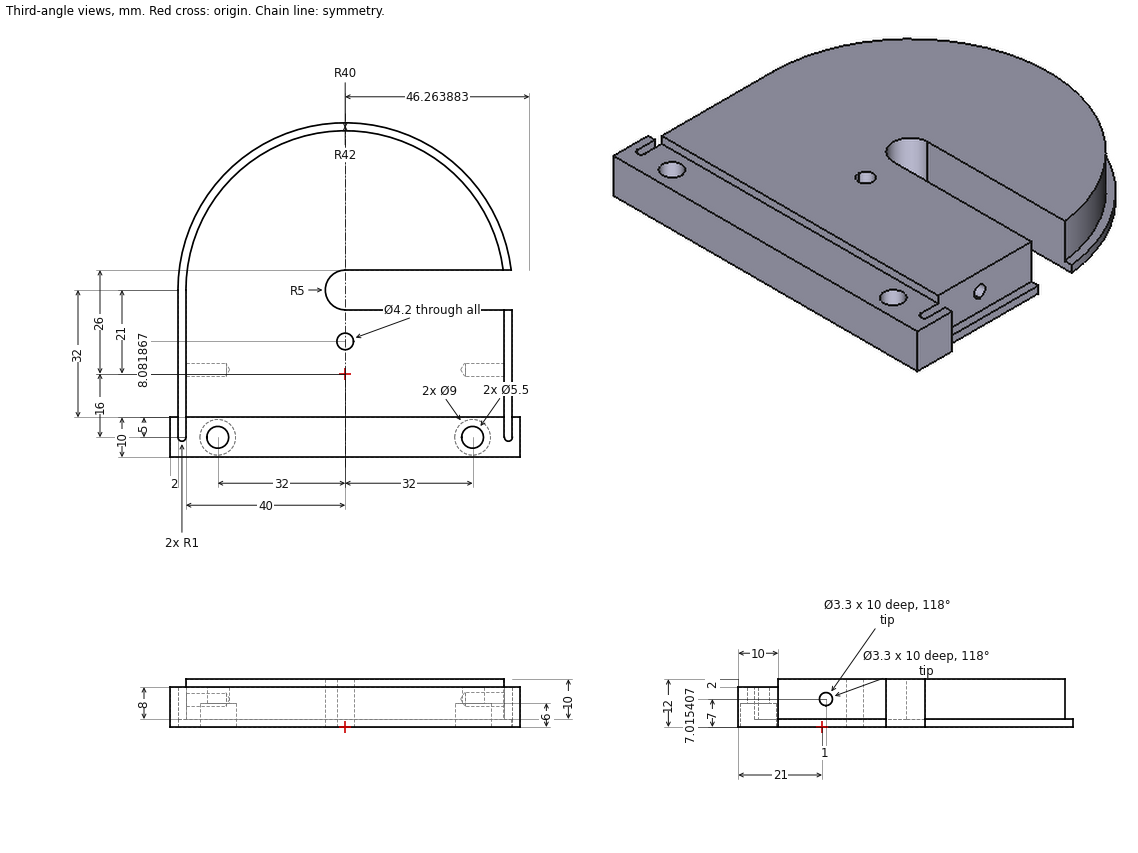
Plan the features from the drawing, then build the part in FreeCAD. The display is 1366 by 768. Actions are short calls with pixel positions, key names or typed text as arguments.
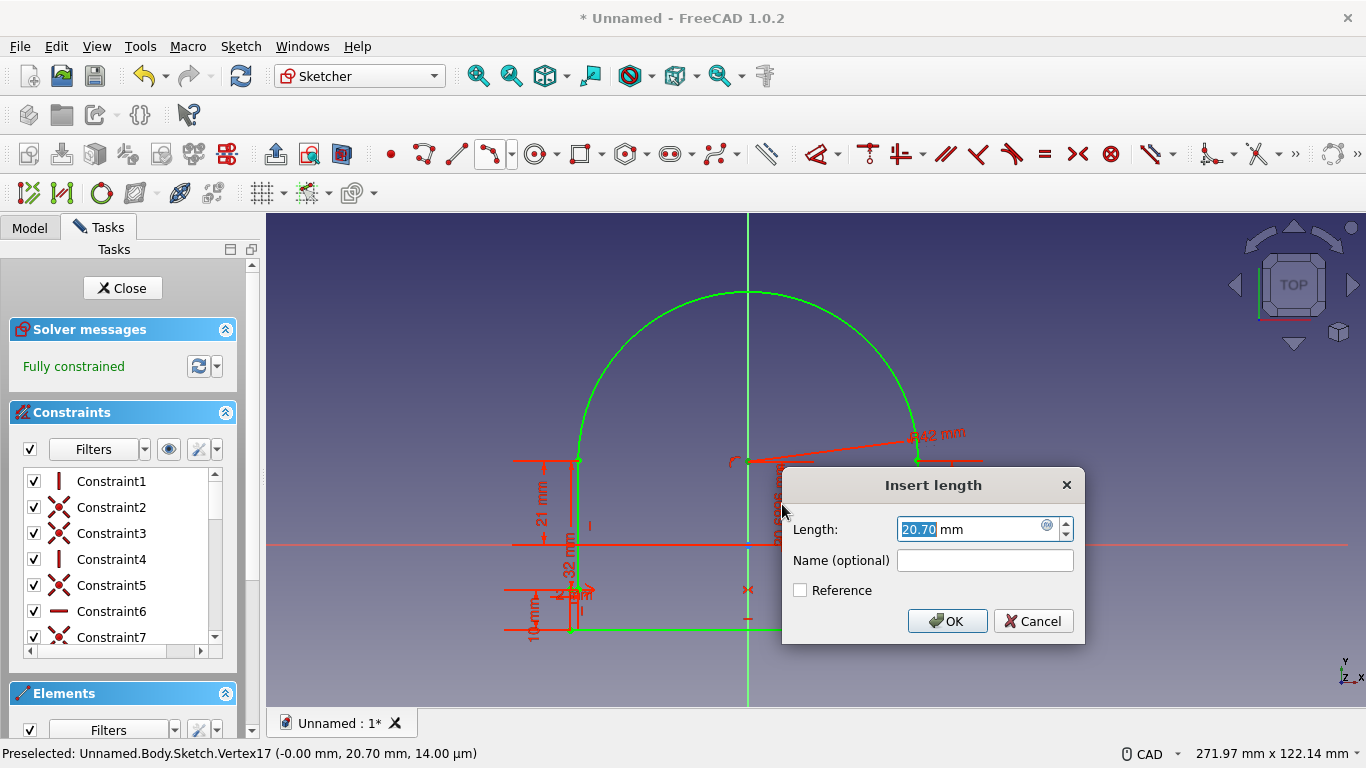
text(21)
key(Return)
key(Escape)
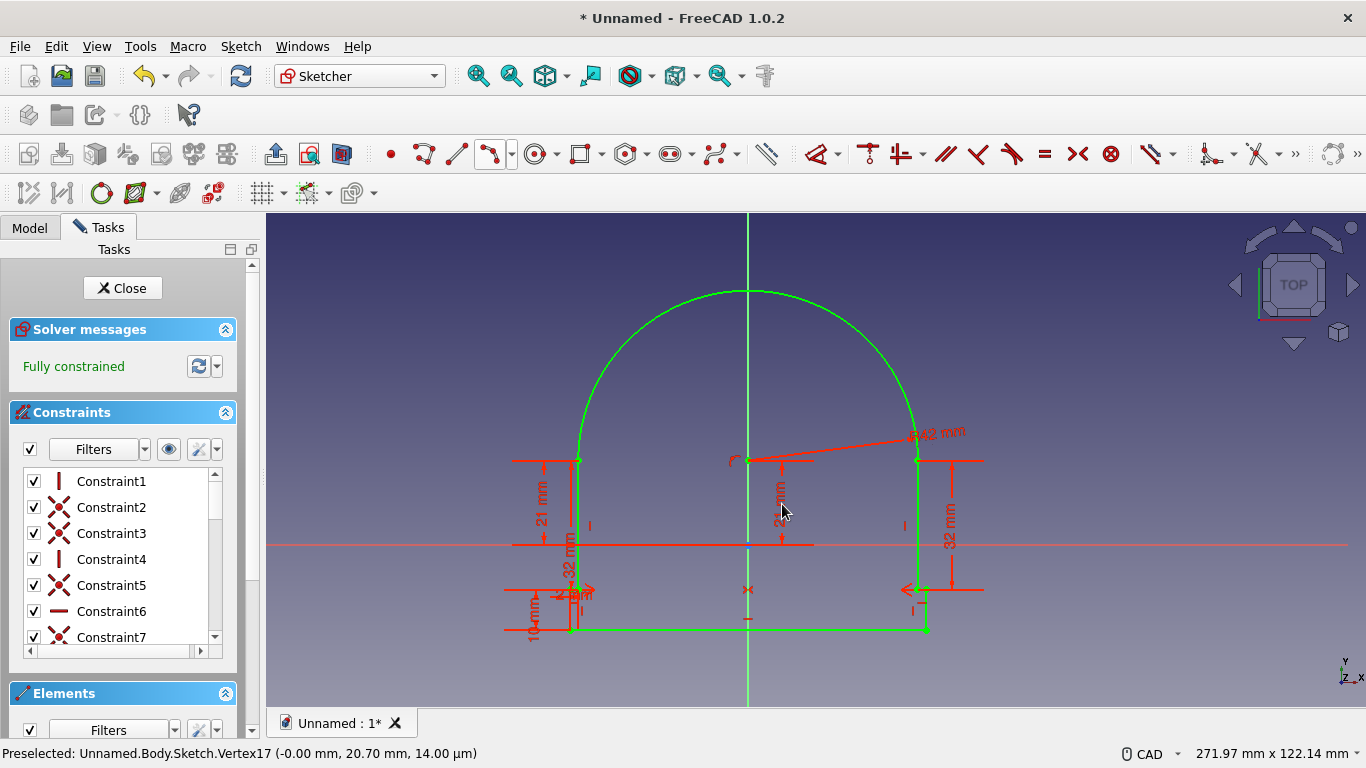
click(123, 288)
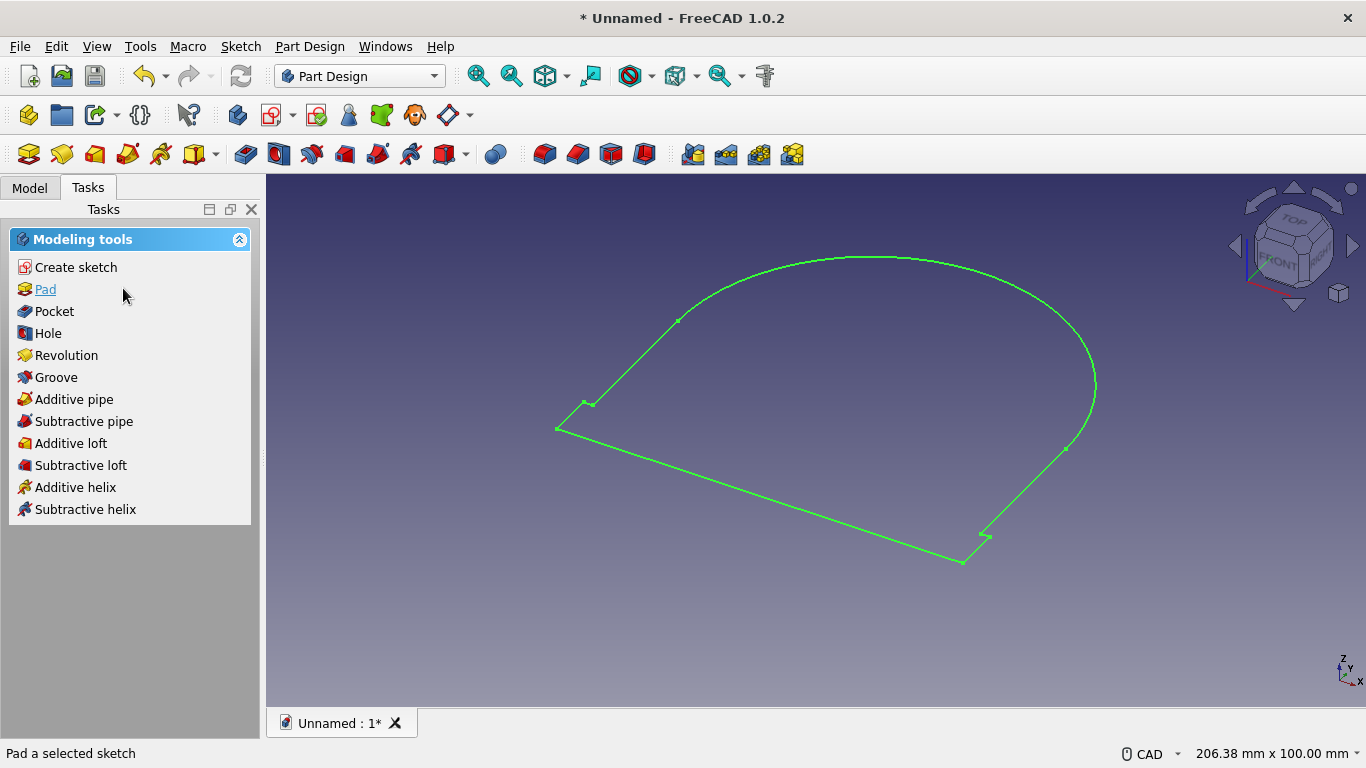
click(29, 154)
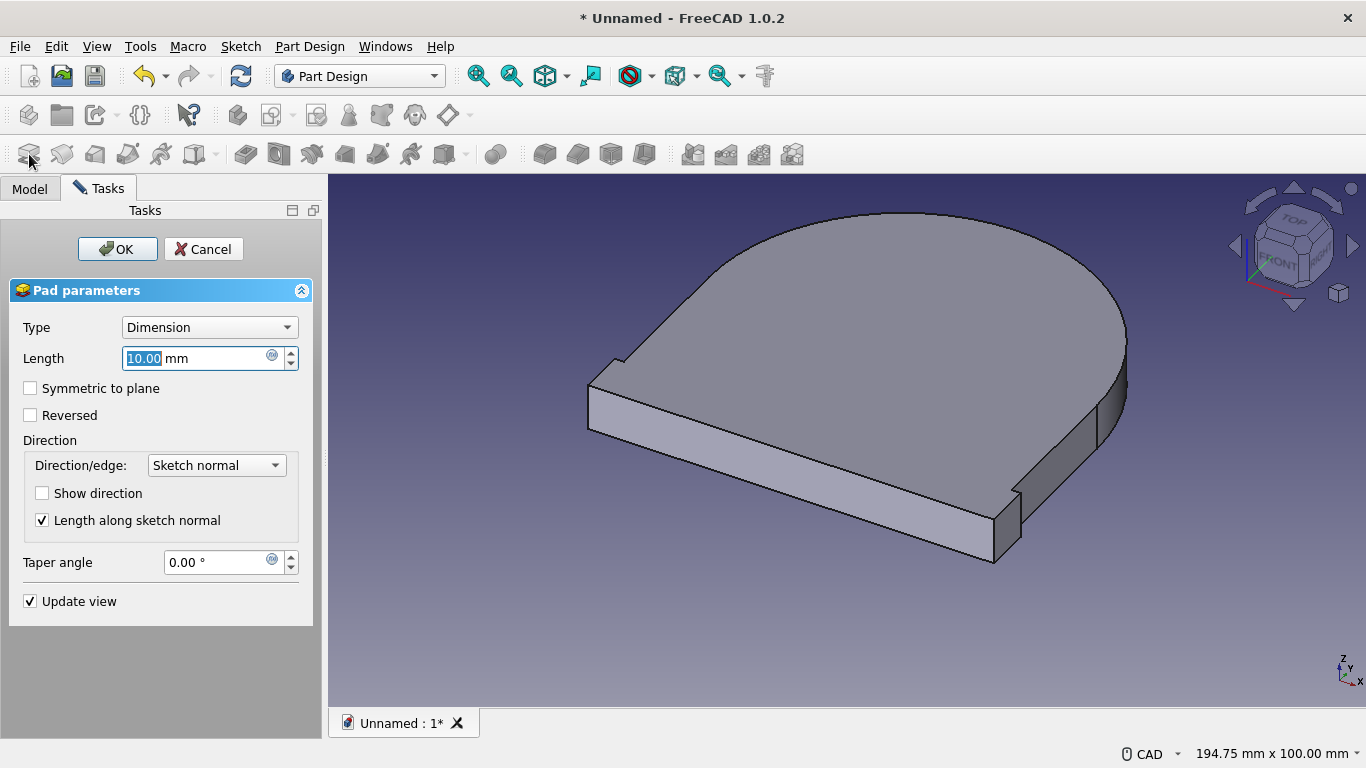
text(12)
key(Tab)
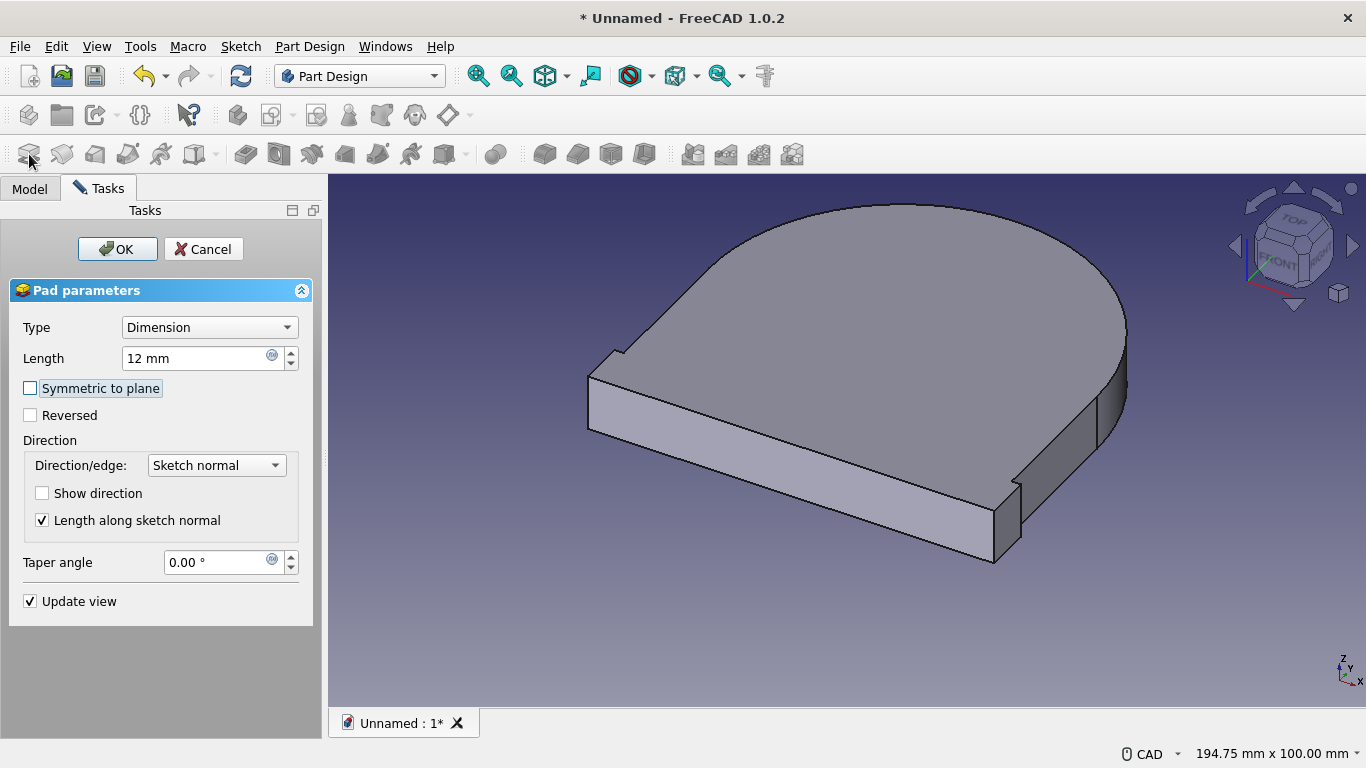
click(118, 249)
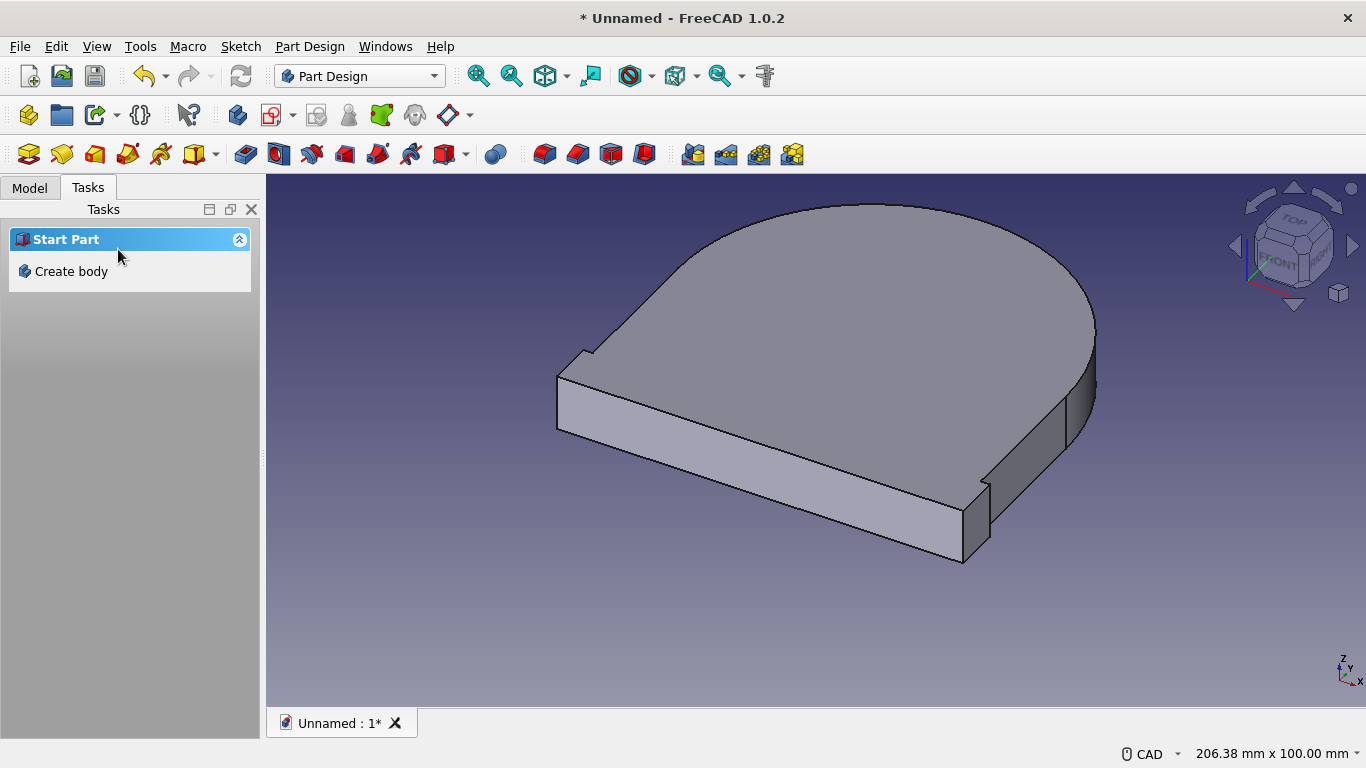
click(479, 76)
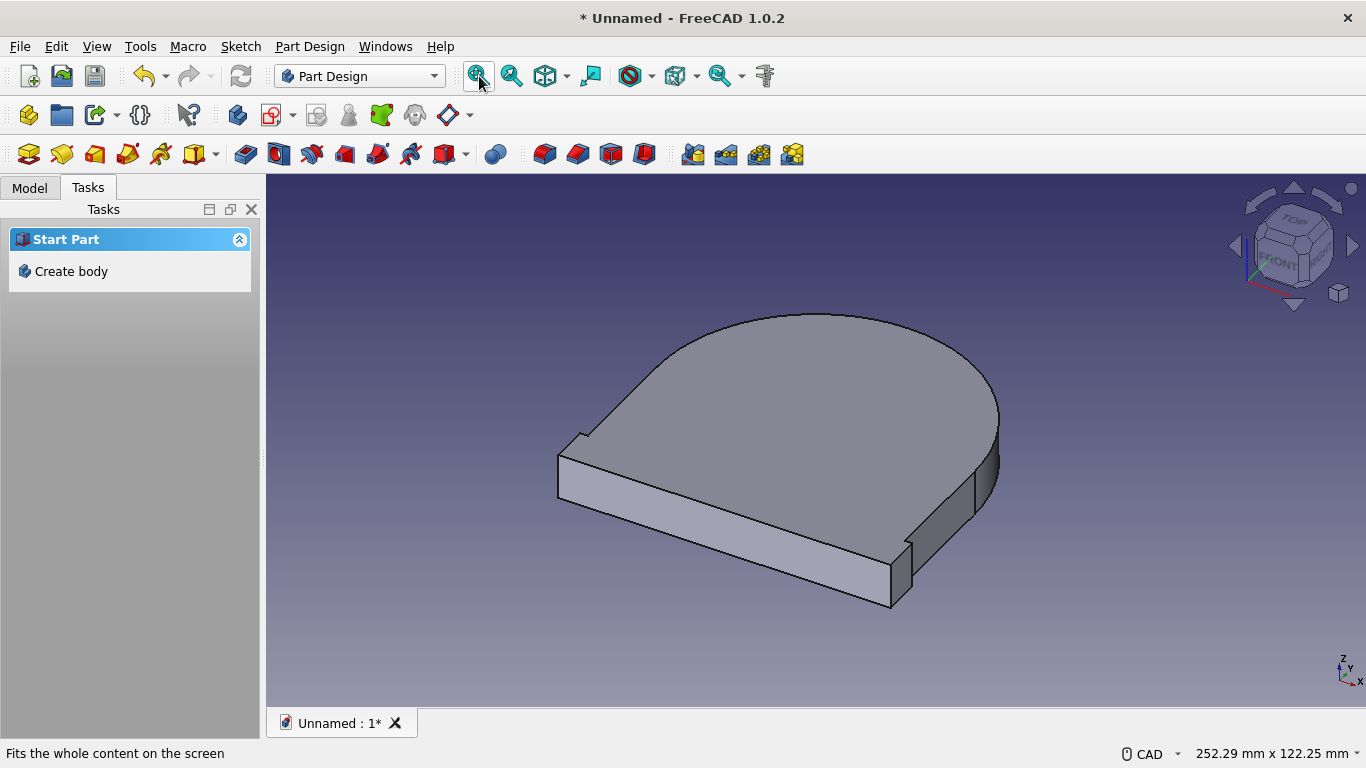
click(30, 188)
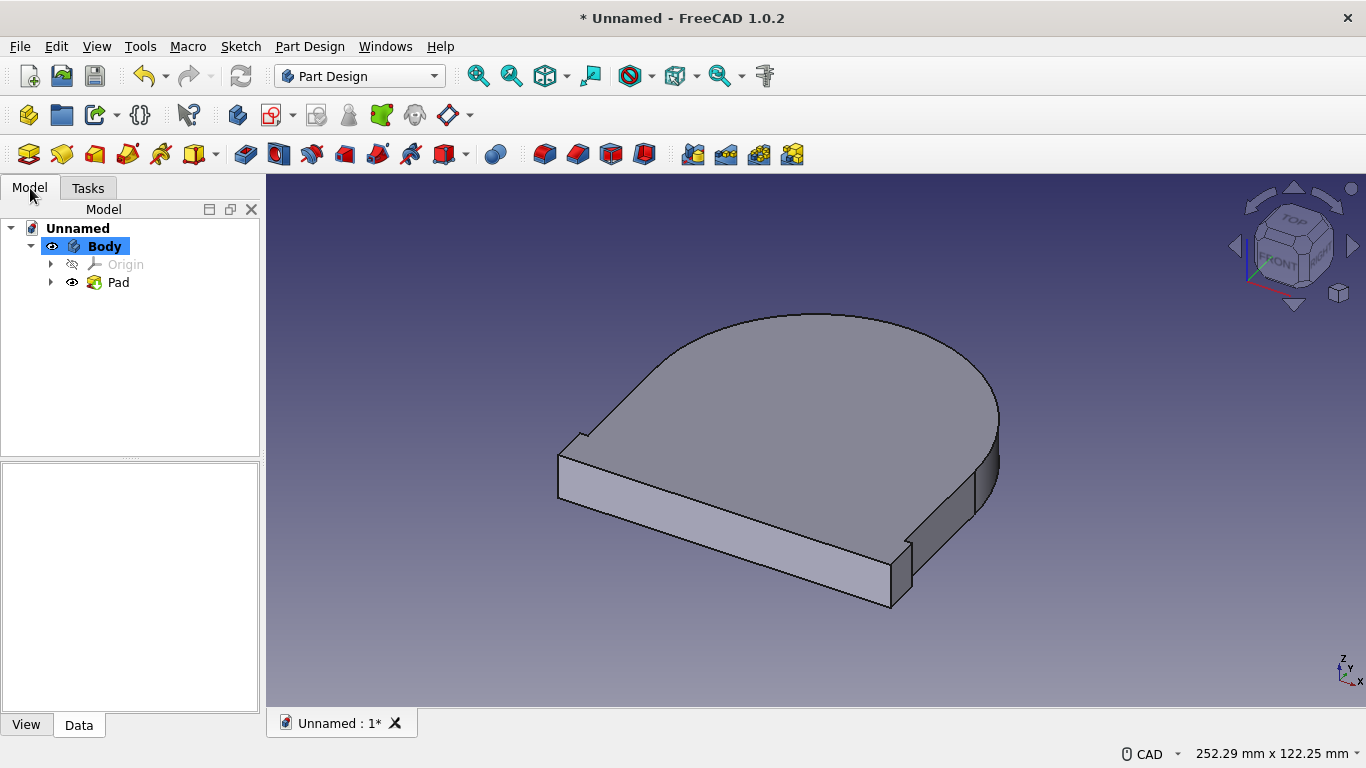
click(51, 264)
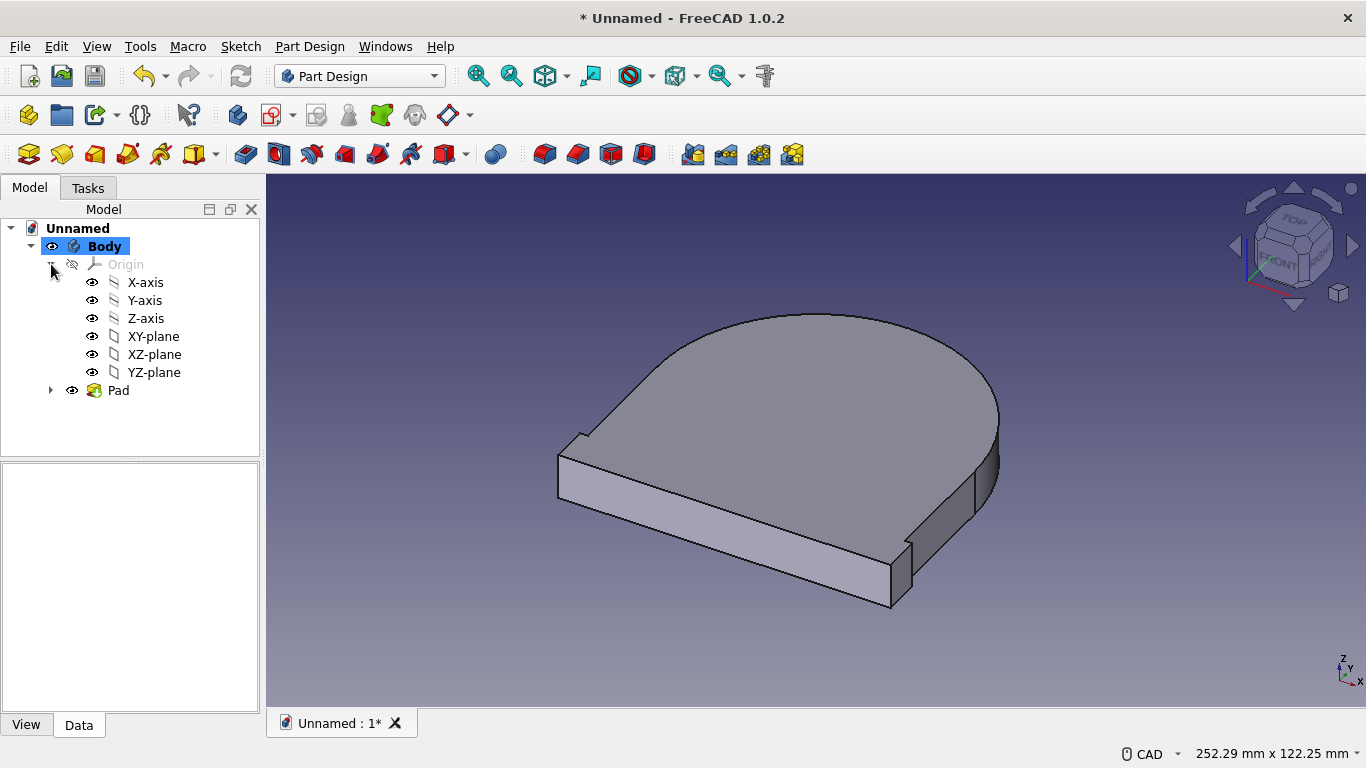
click(137, 336)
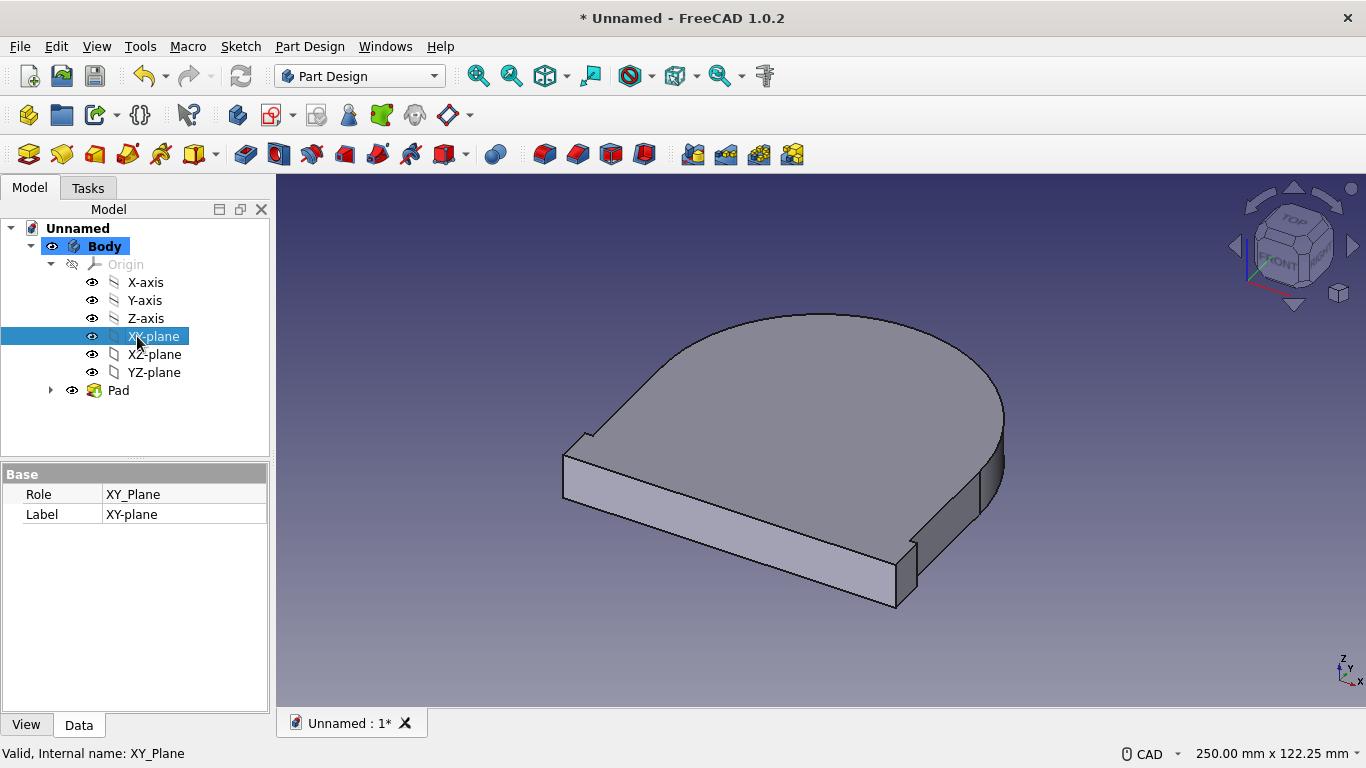
click(448, 116)